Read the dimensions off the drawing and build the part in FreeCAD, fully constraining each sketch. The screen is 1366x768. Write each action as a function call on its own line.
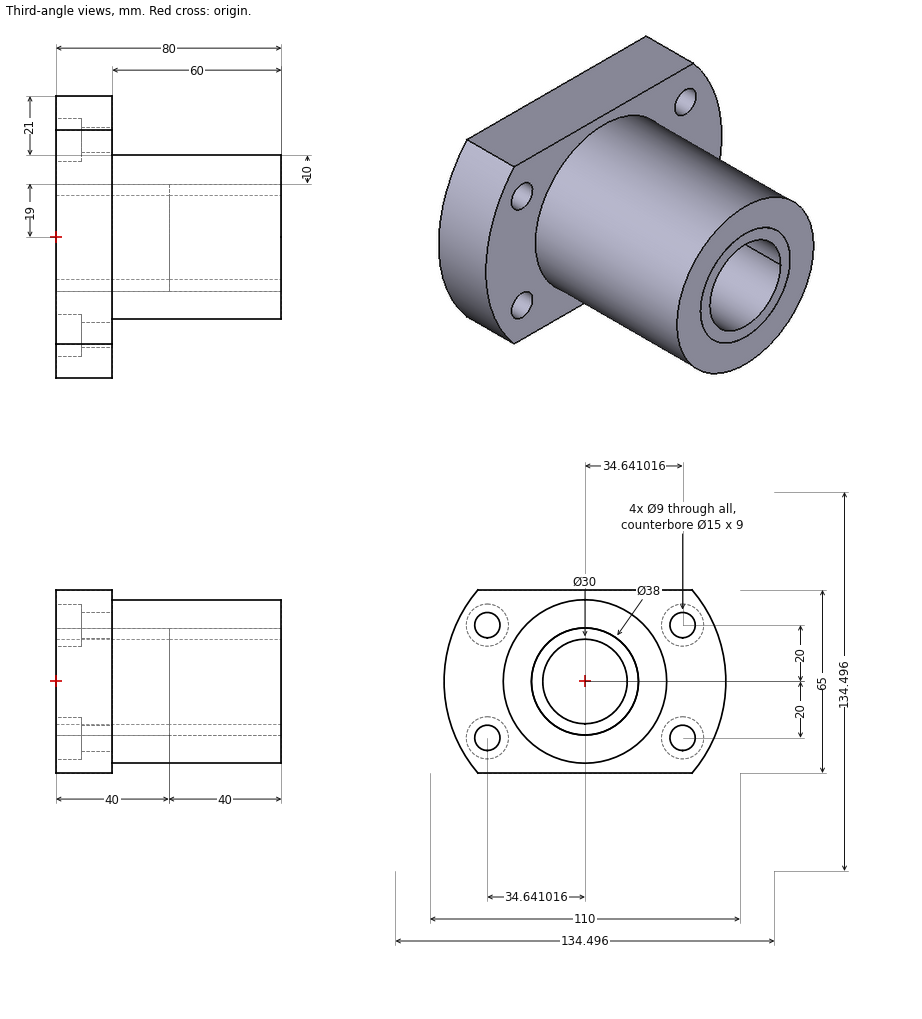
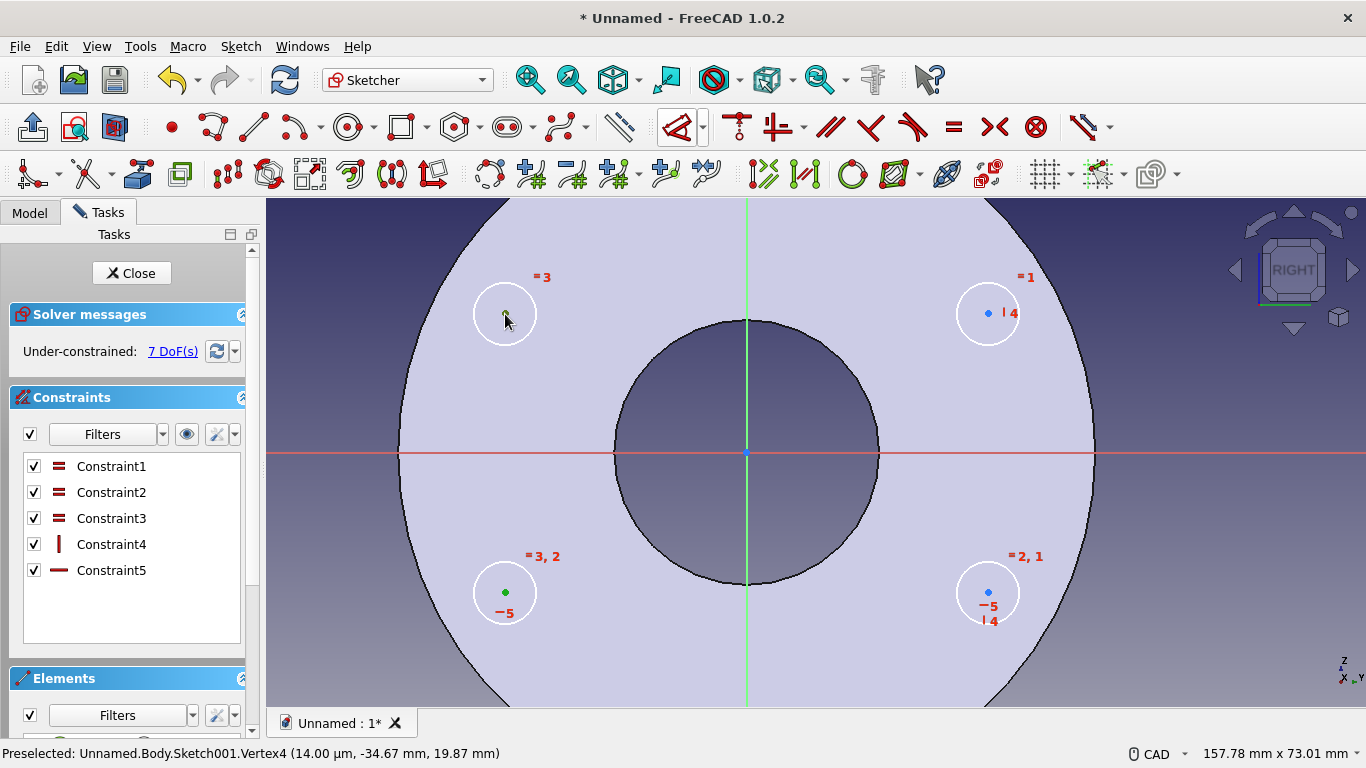
click(804, 128)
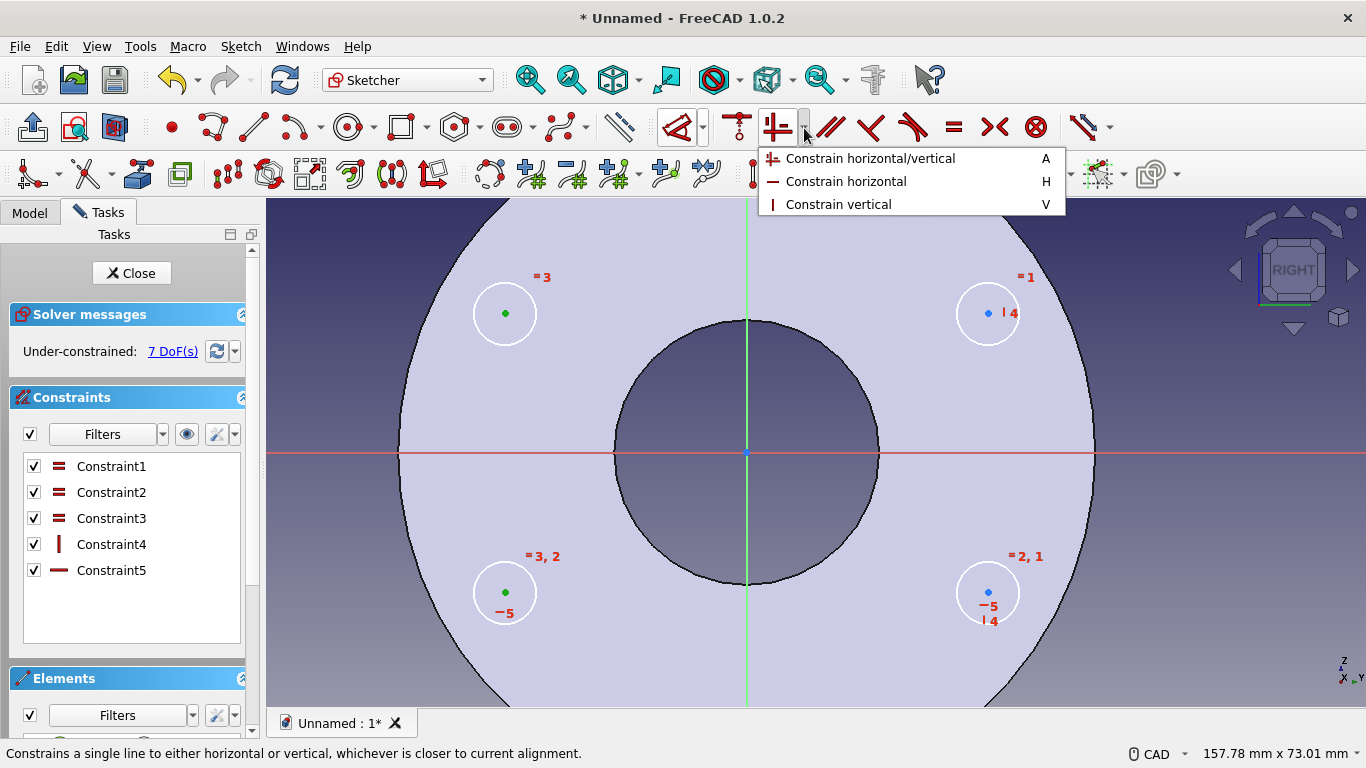
click(912, 204)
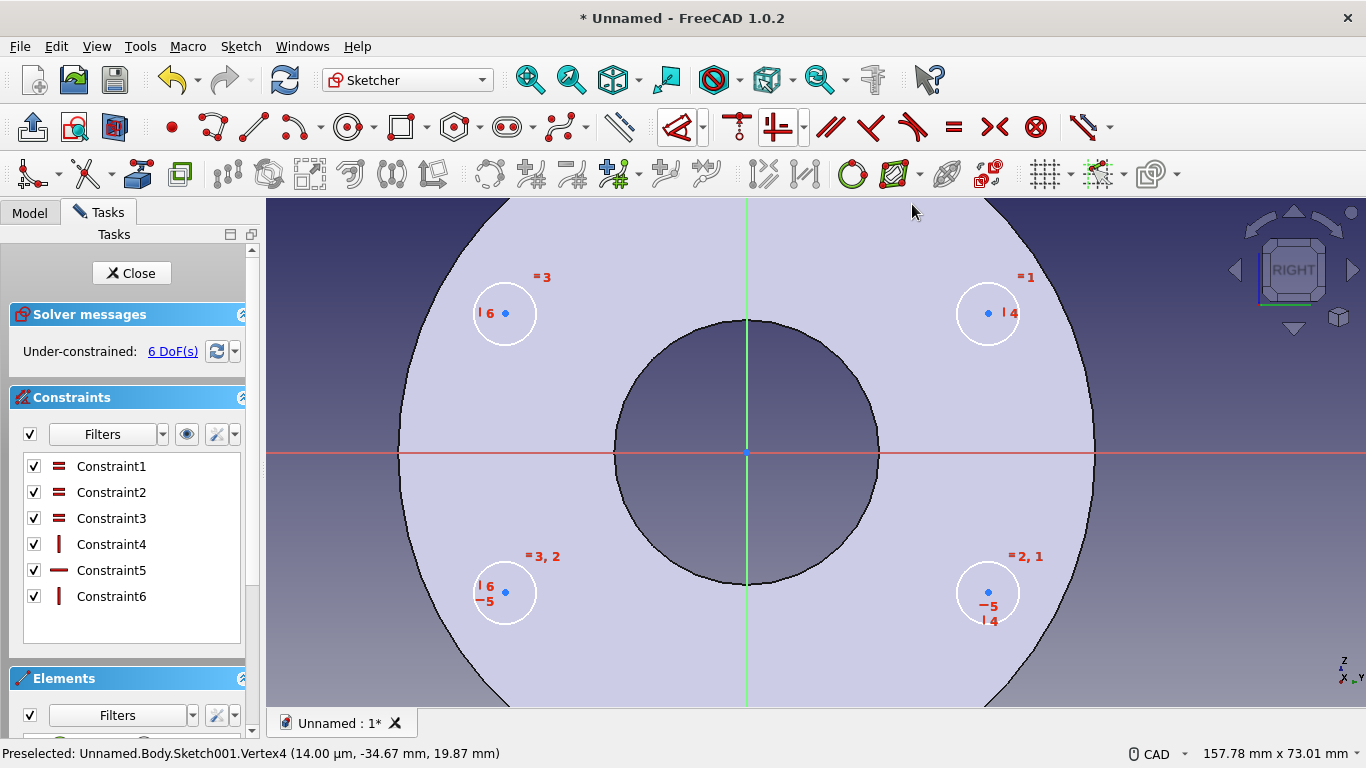
click(988, 314)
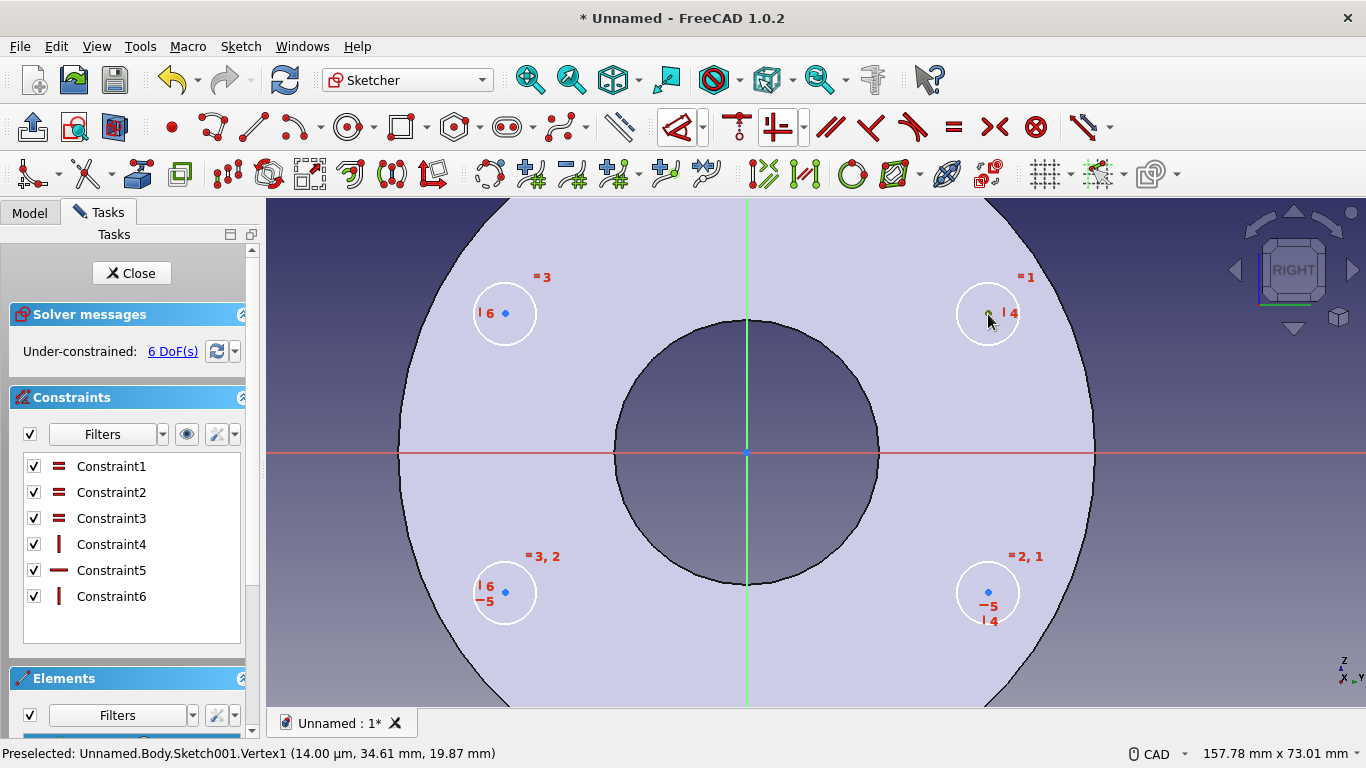
click(505, 314)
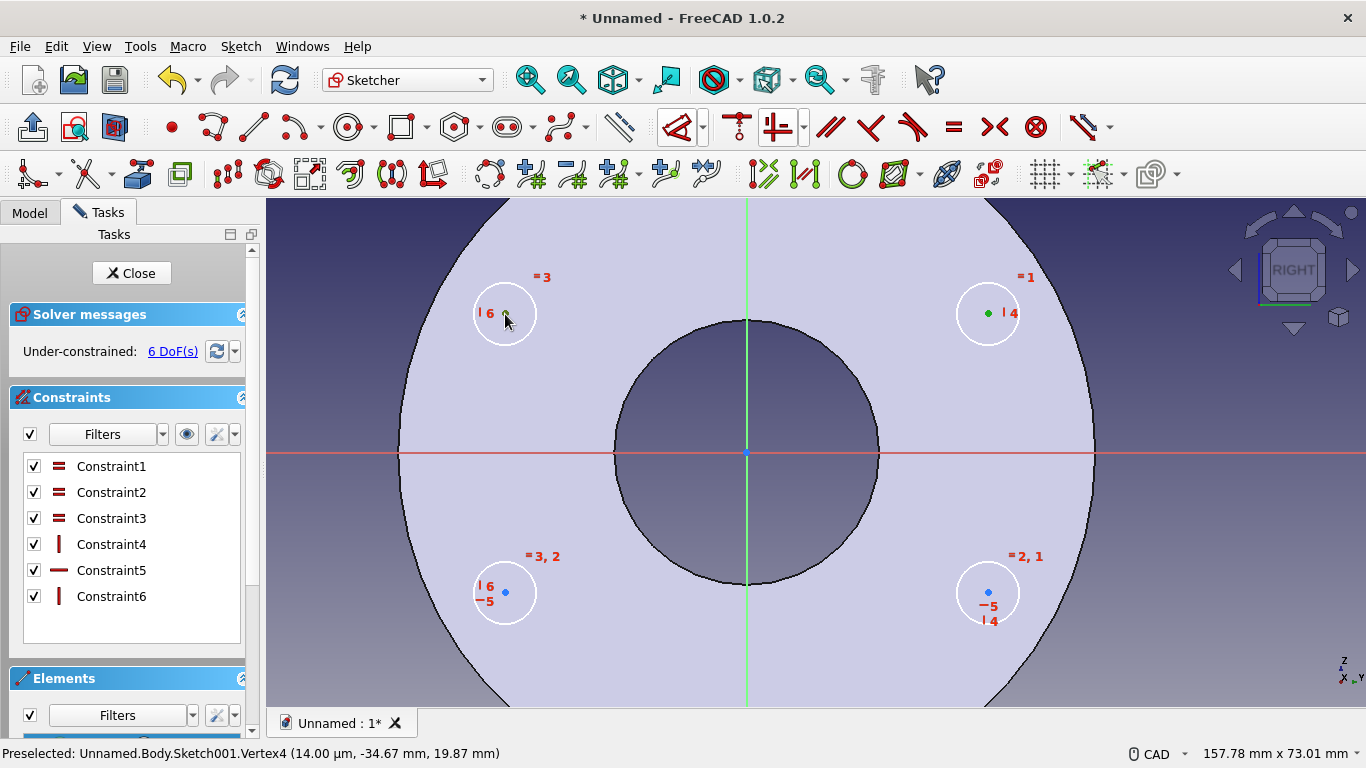
key(h)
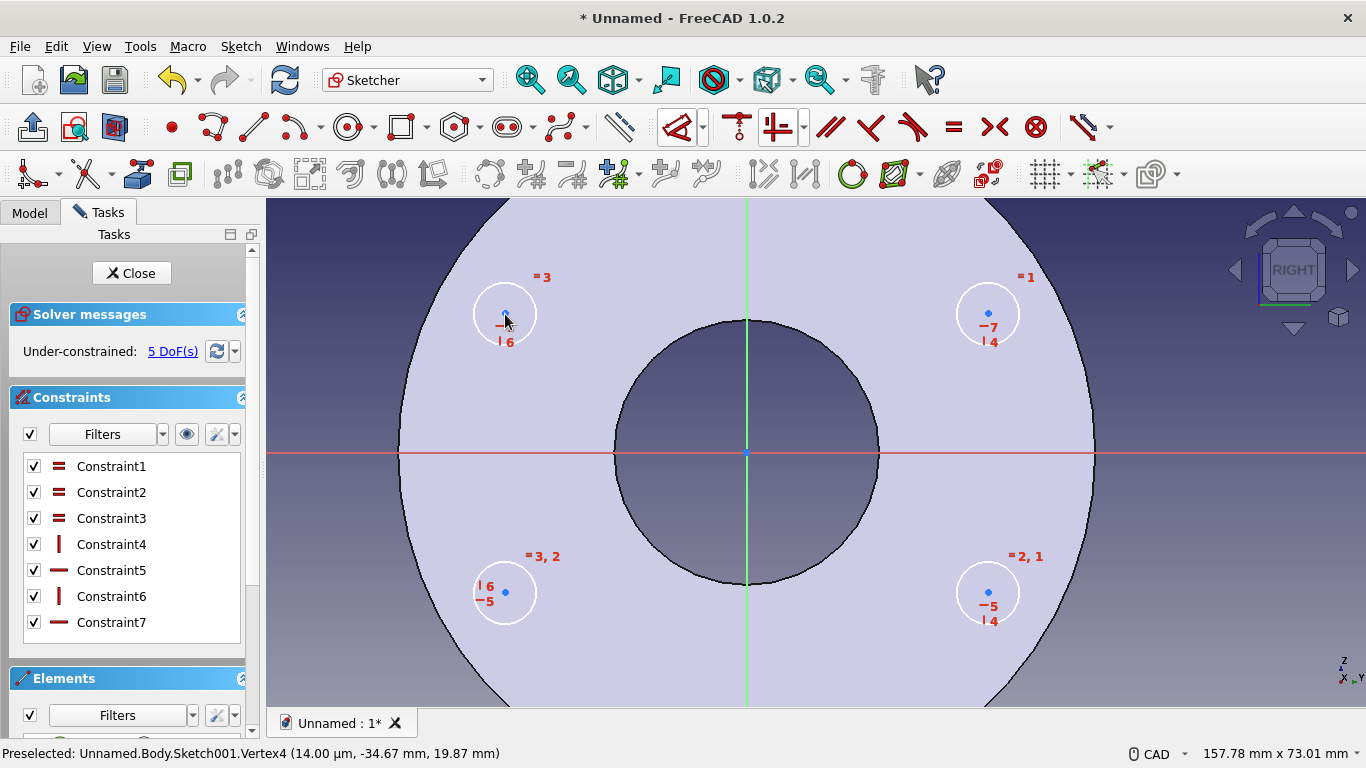
click(676, 128)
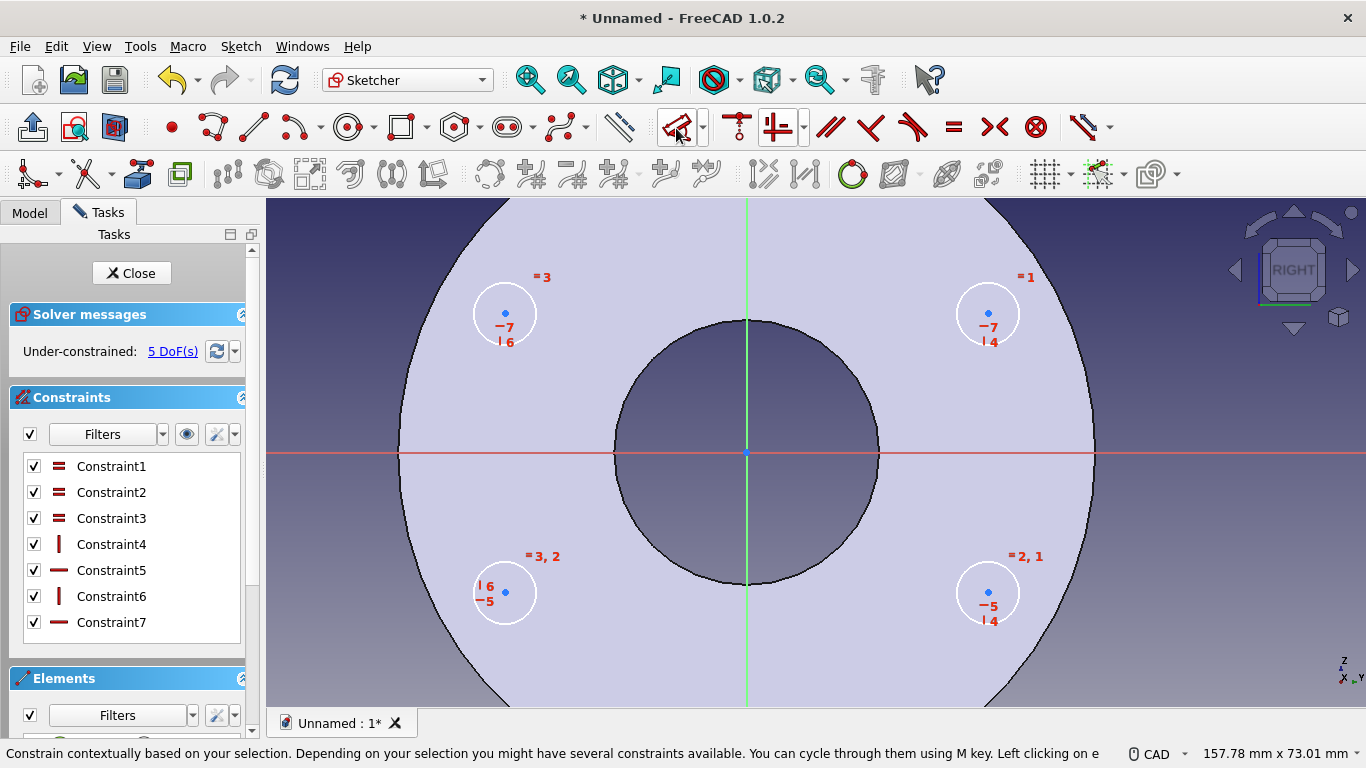
click(1010, 292)
click(1033, 269)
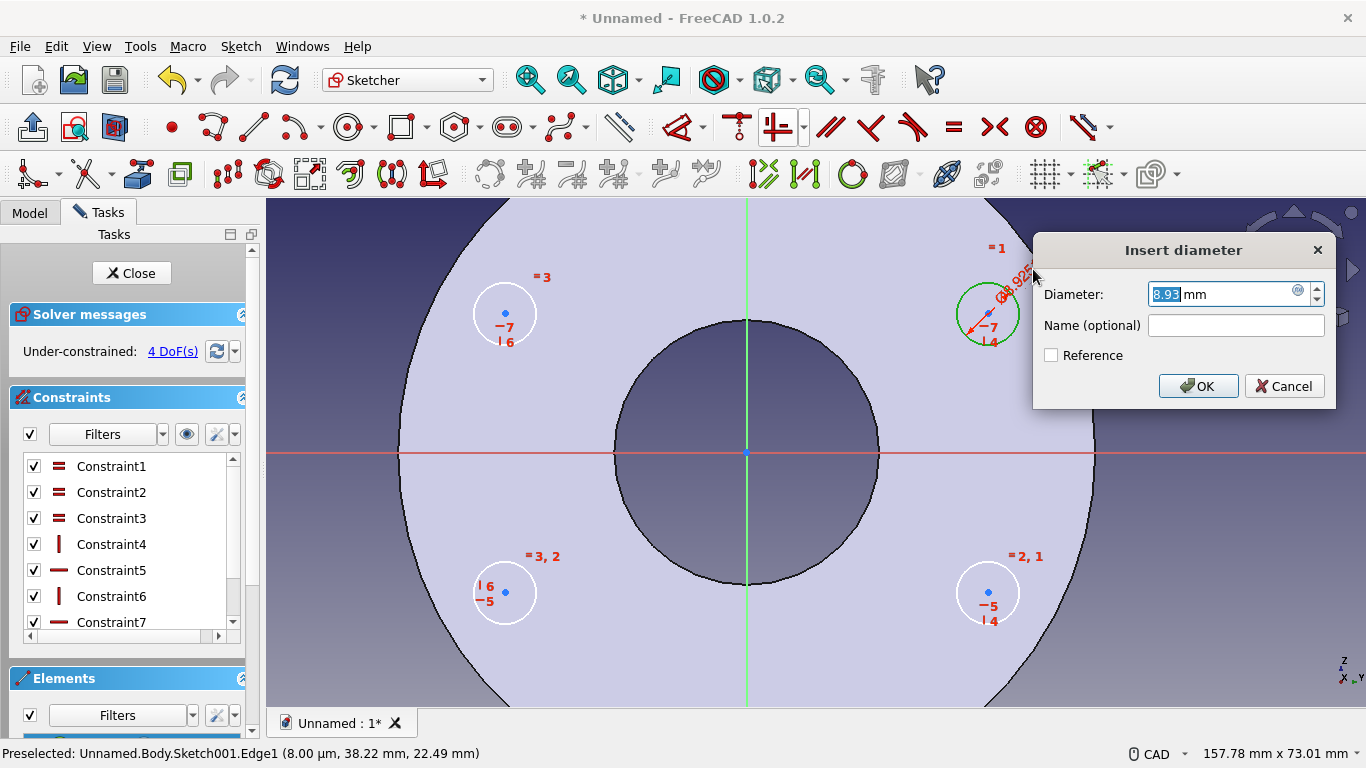
text(9)
key(Return)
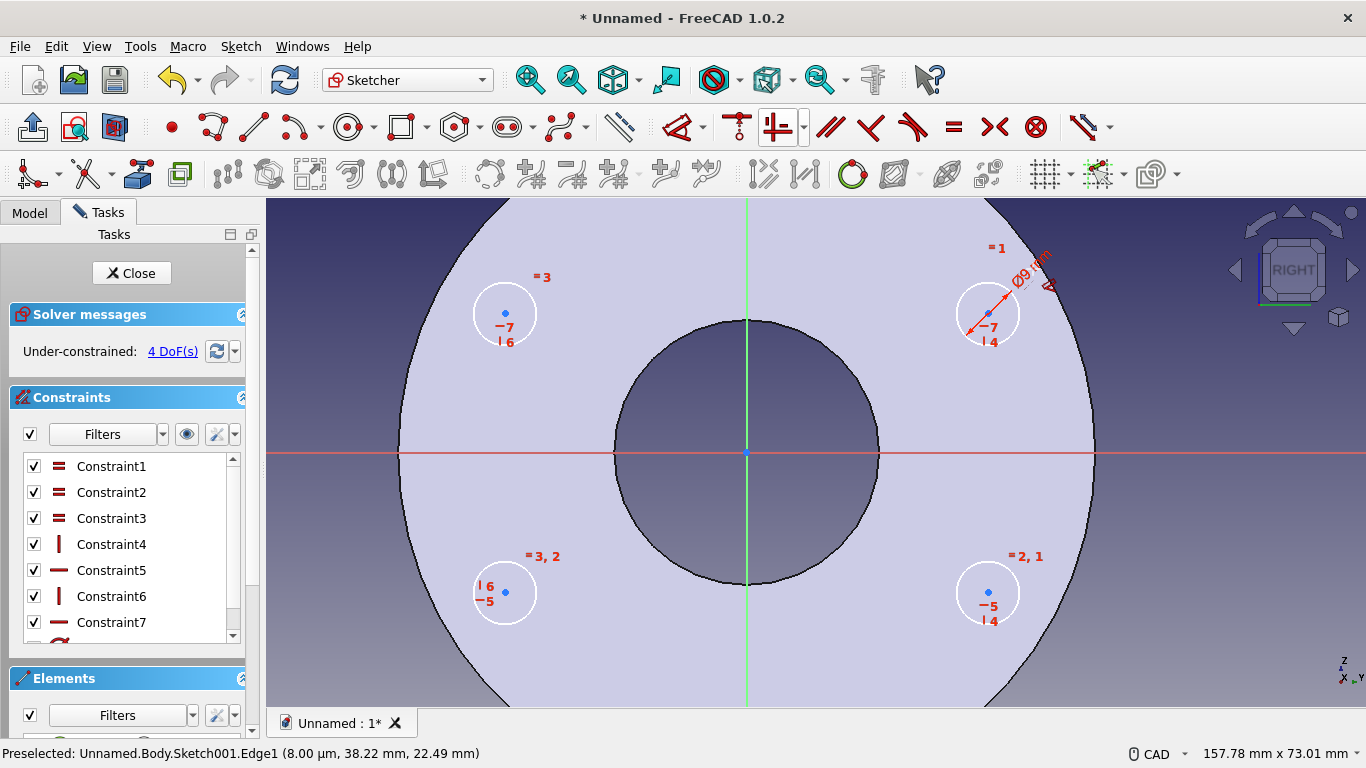
click(988, 314)
click(1022, 383)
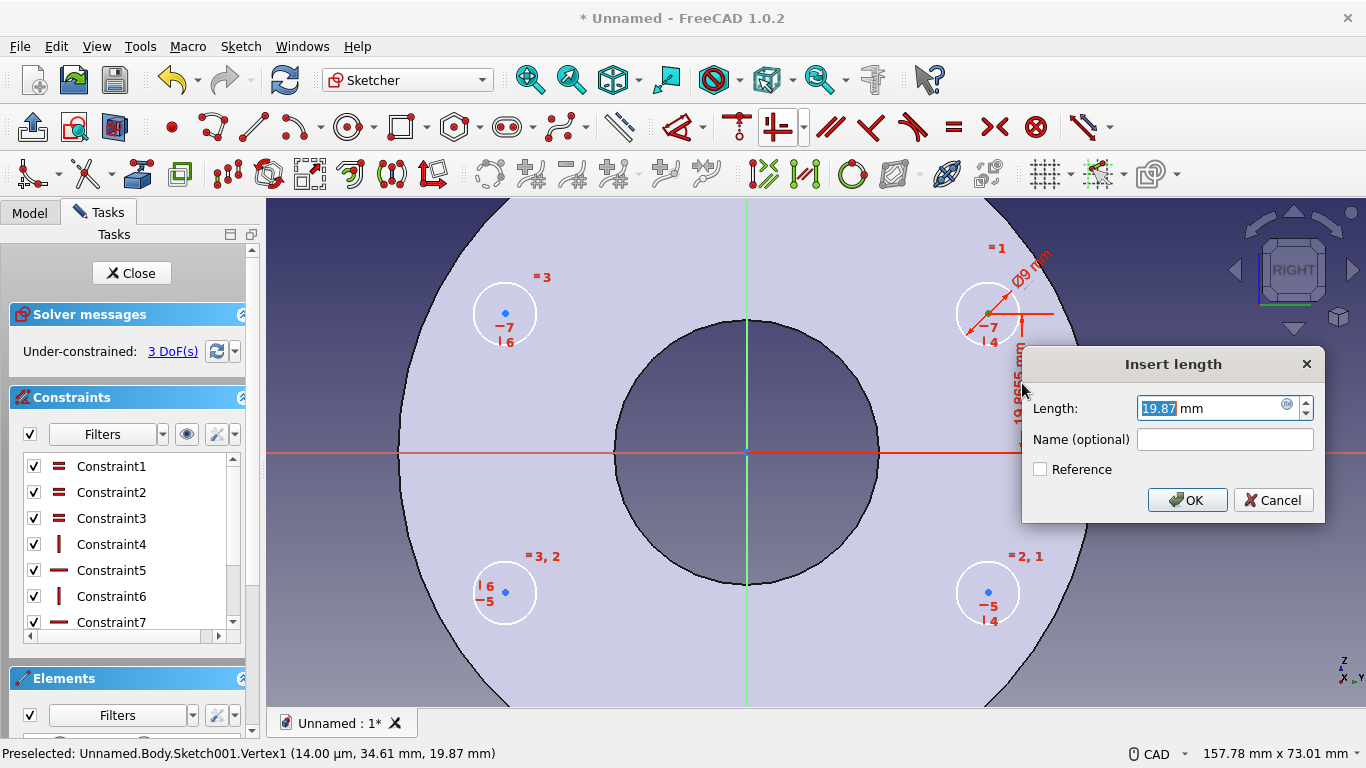
text(20)
key(Return)